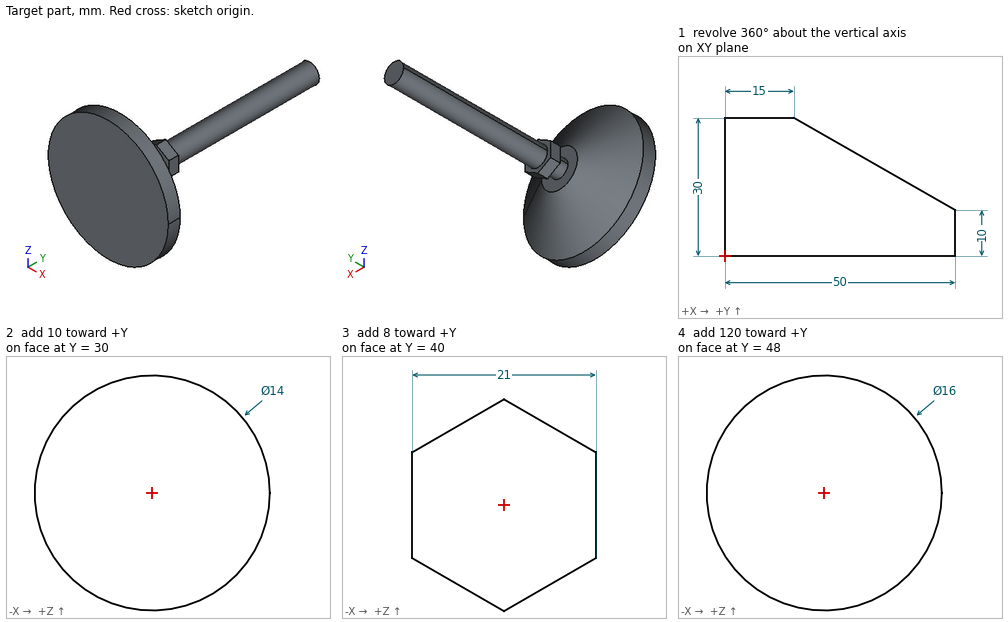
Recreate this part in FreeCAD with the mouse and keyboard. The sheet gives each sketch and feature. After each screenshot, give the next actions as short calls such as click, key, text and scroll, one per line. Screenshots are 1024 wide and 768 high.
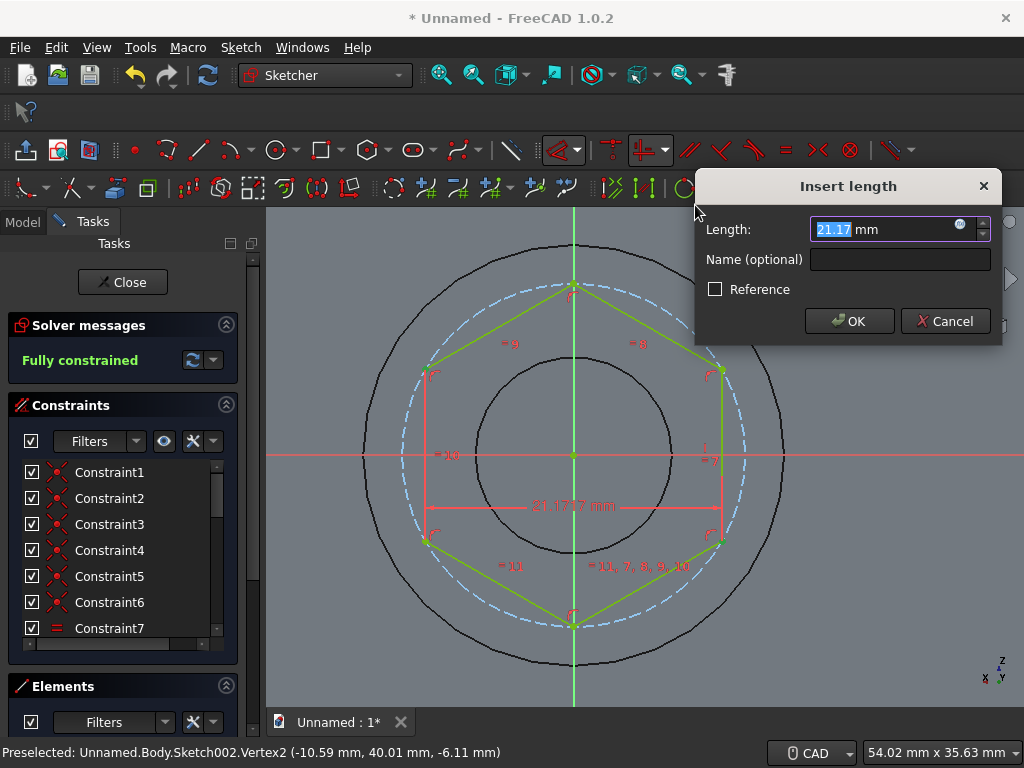
text(21)
key(Return)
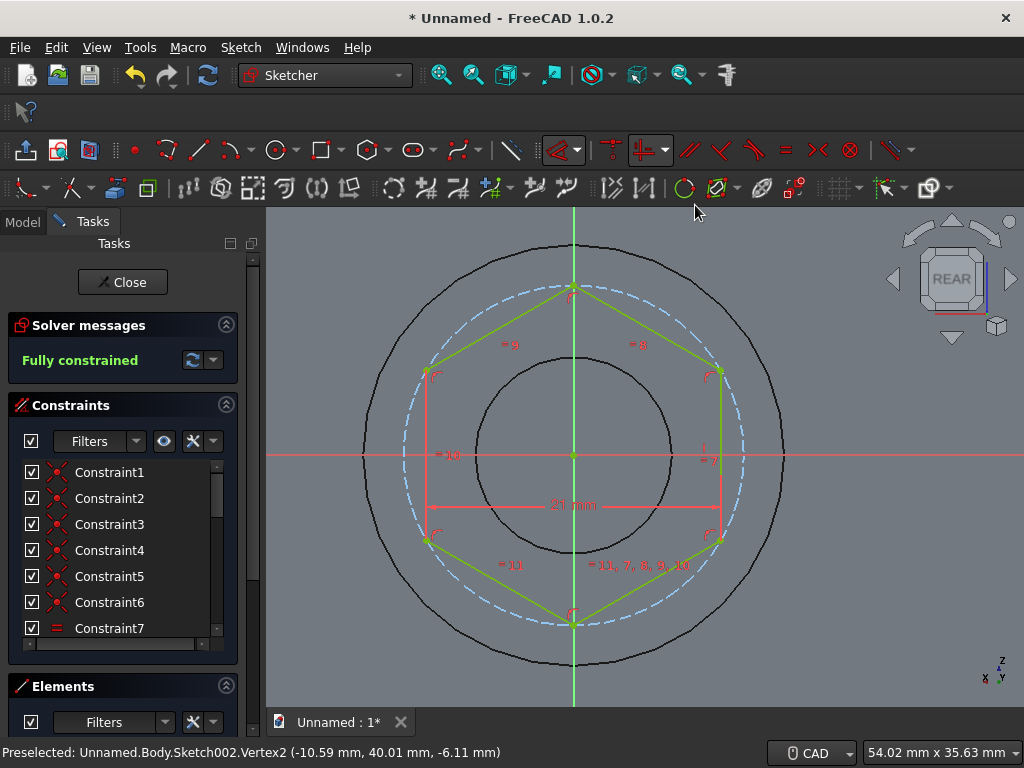
click(123, 282)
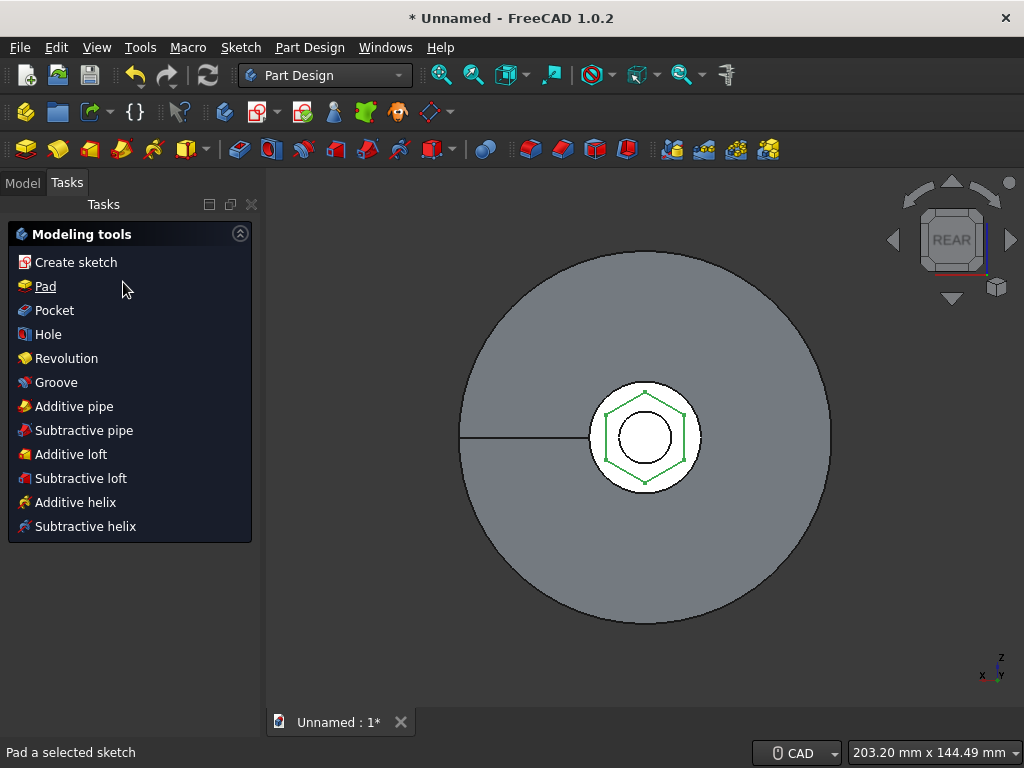
click(26, 150)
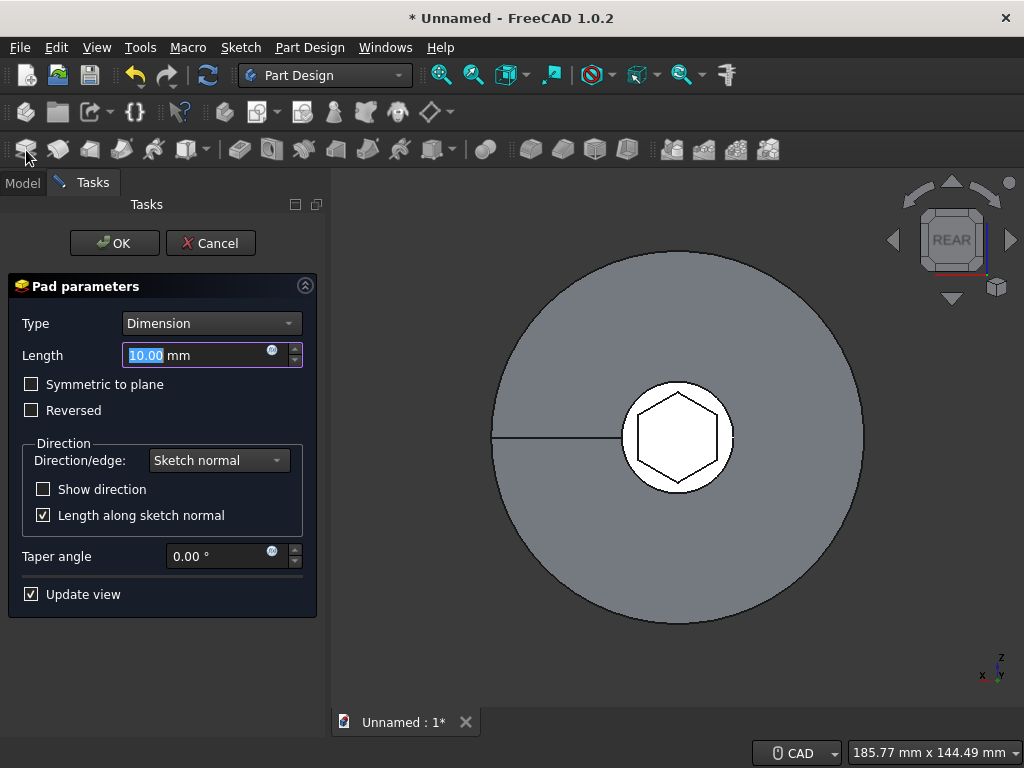
text(8)
key(Tab)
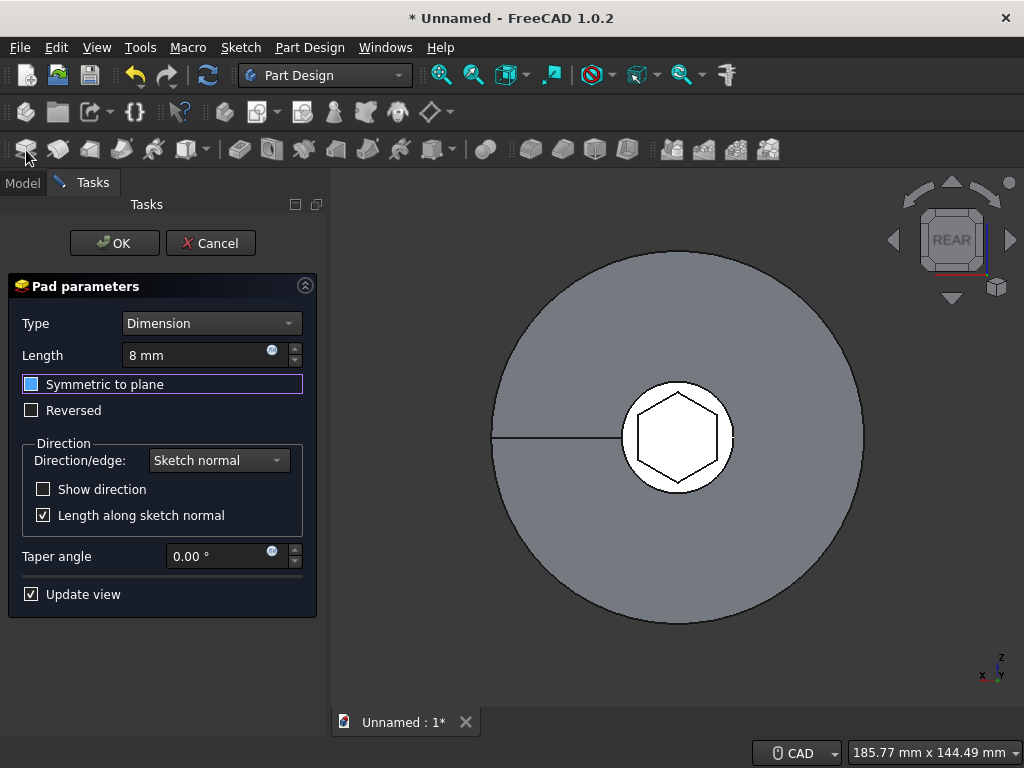
click(115, 243)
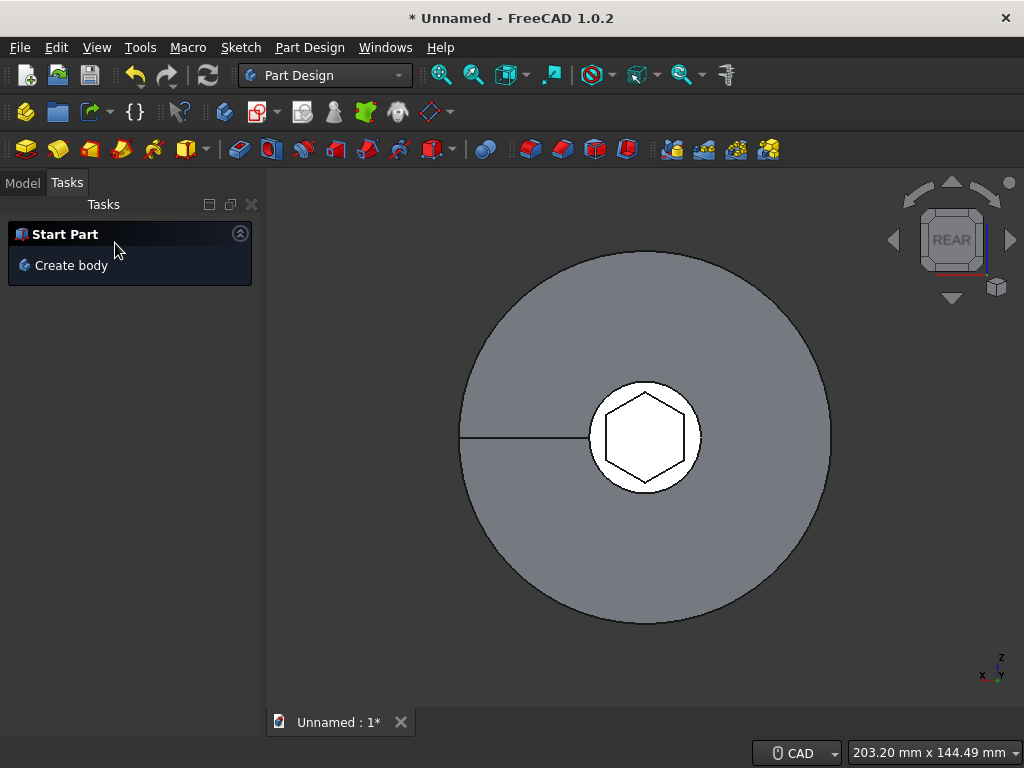
click(645, 436)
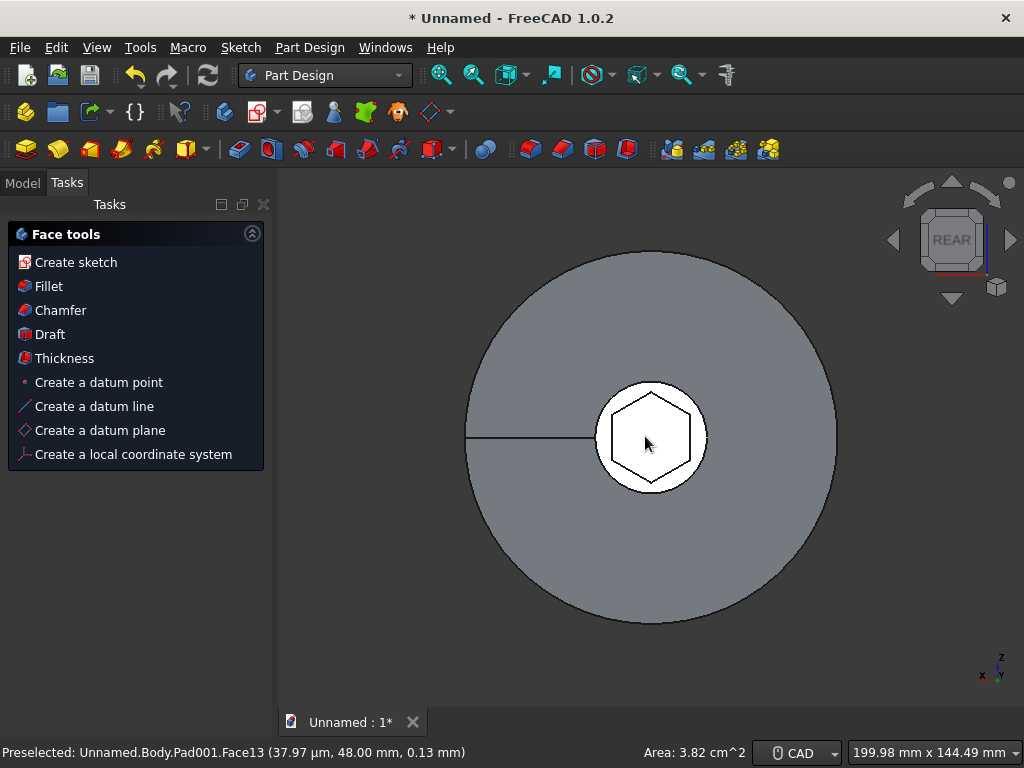
click(258, 112)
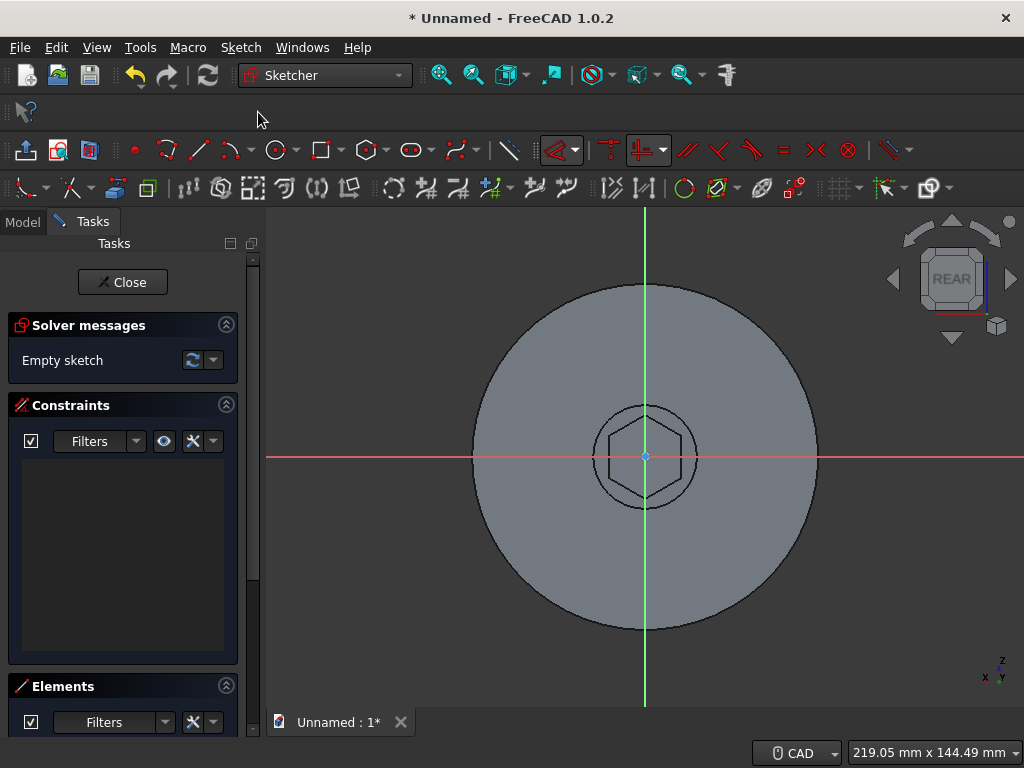
scroll(659, 457, up, 9)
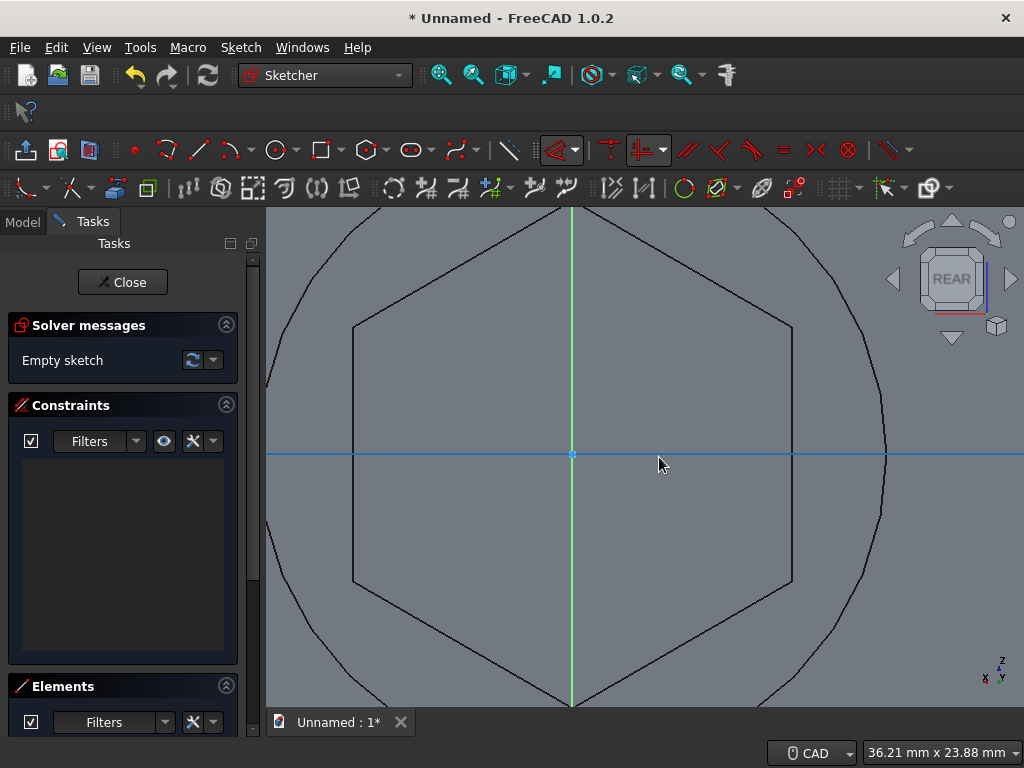
key(g)
key(c)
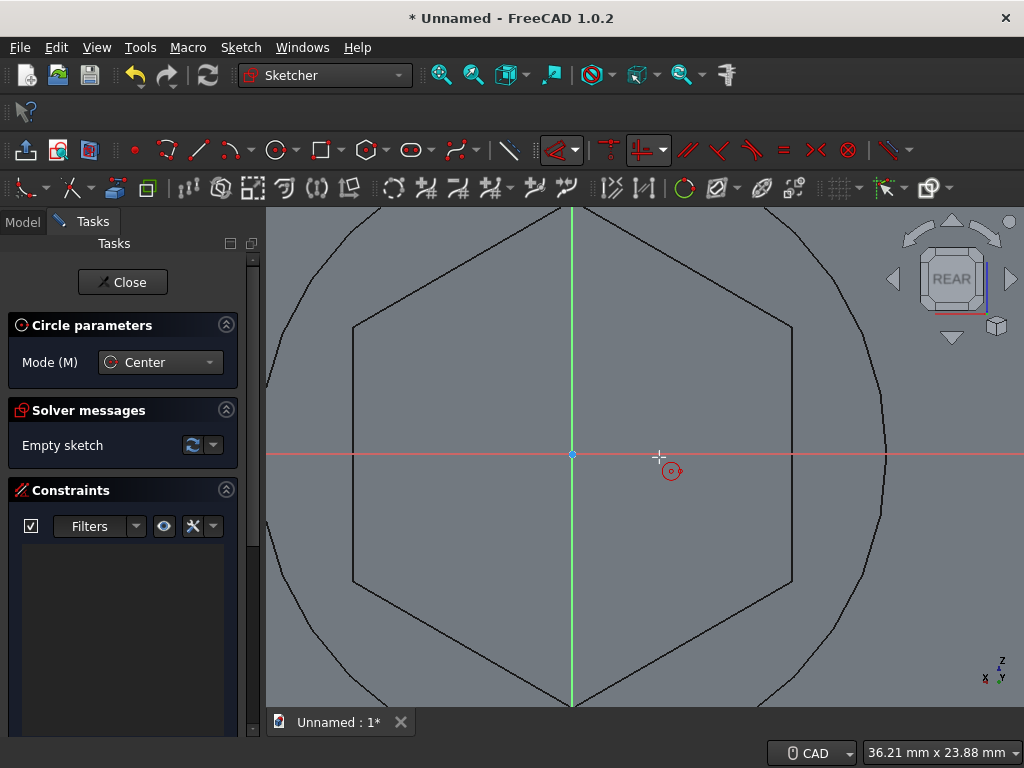
click(572, 454)
move(691, 336)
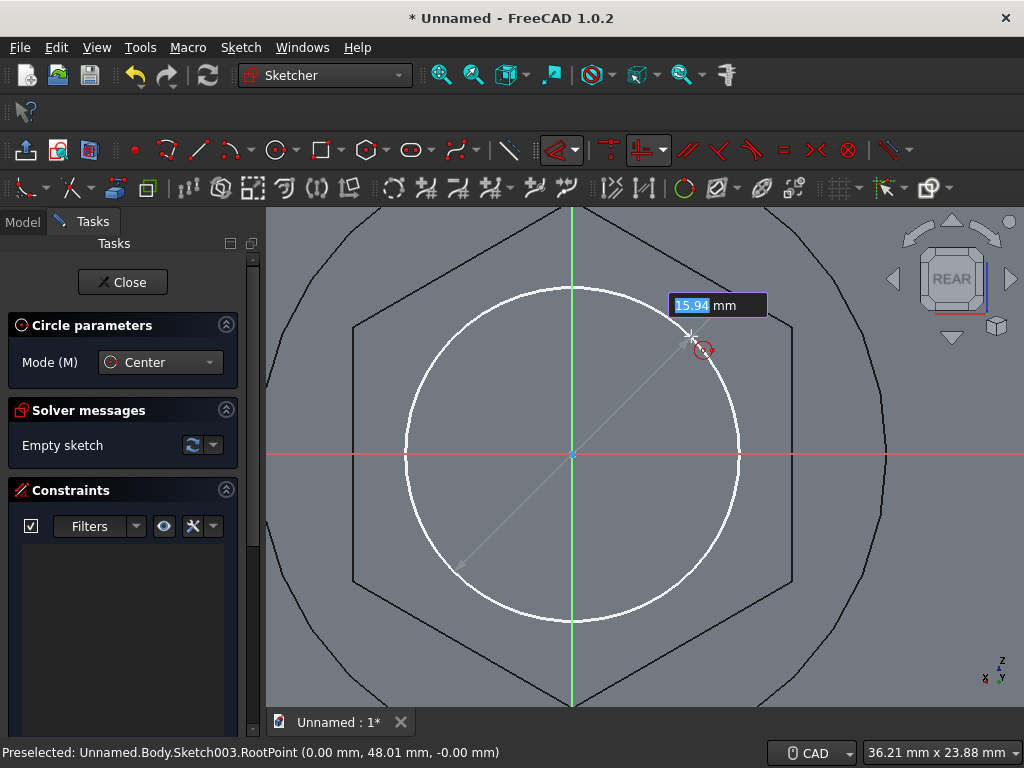
text(16)
key(Return)
key(Escape)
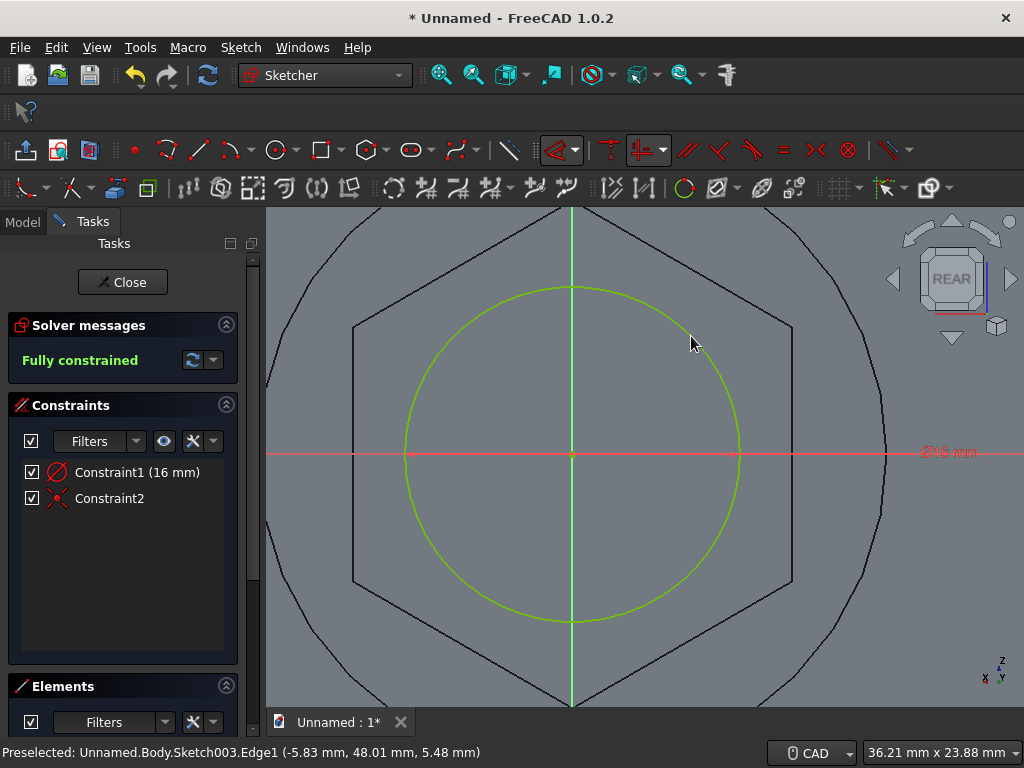
click(123, 282)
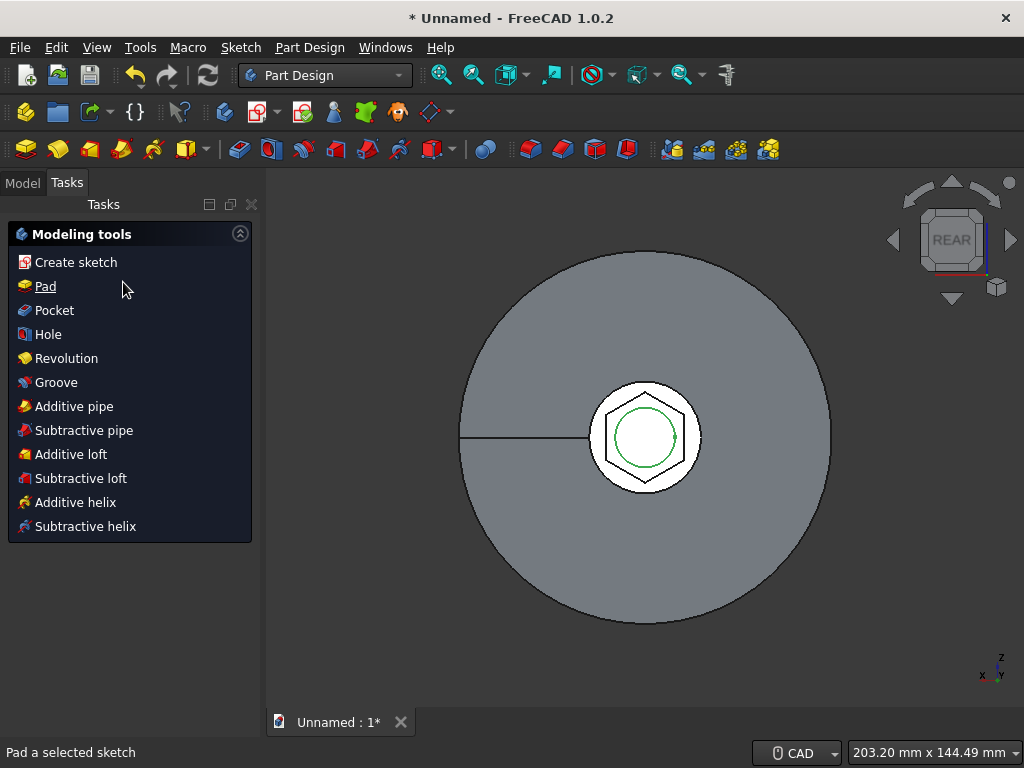
click(26, 150)